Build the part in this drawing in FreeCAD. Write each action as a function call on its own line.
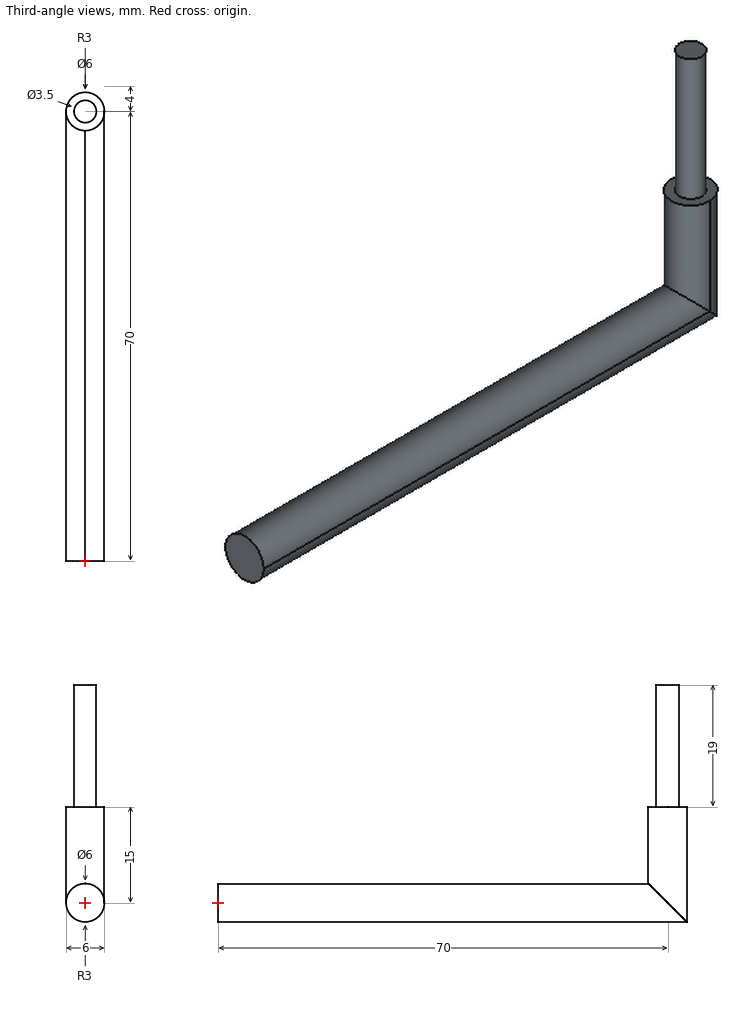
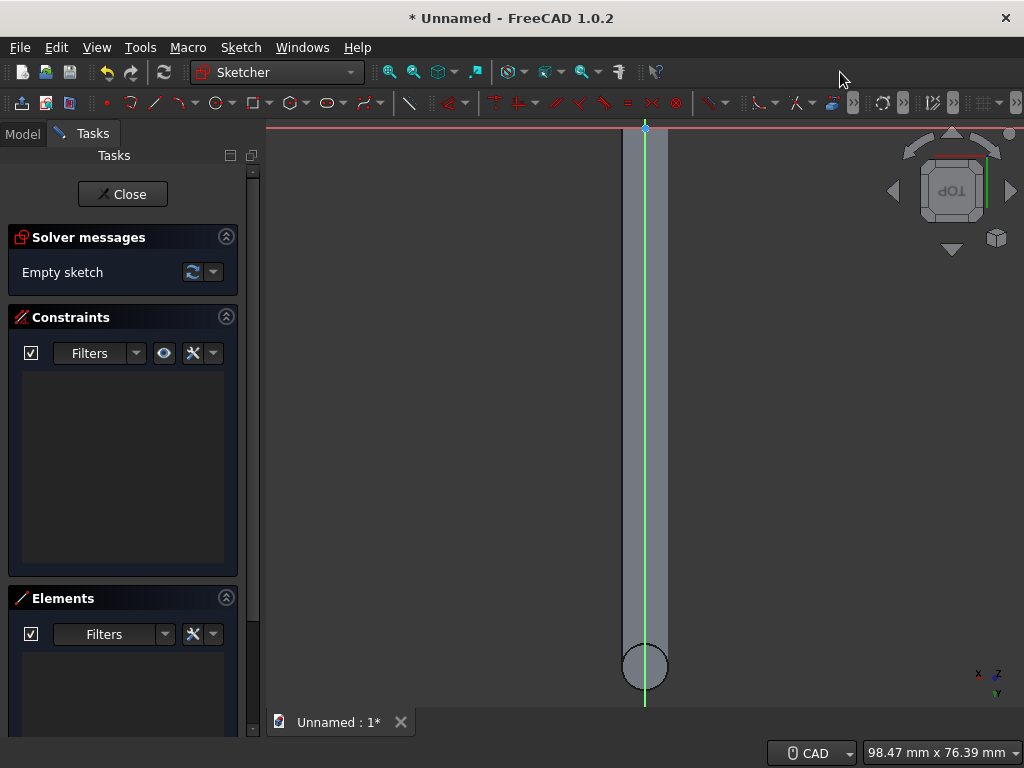
scroll(576, 413, down, 5)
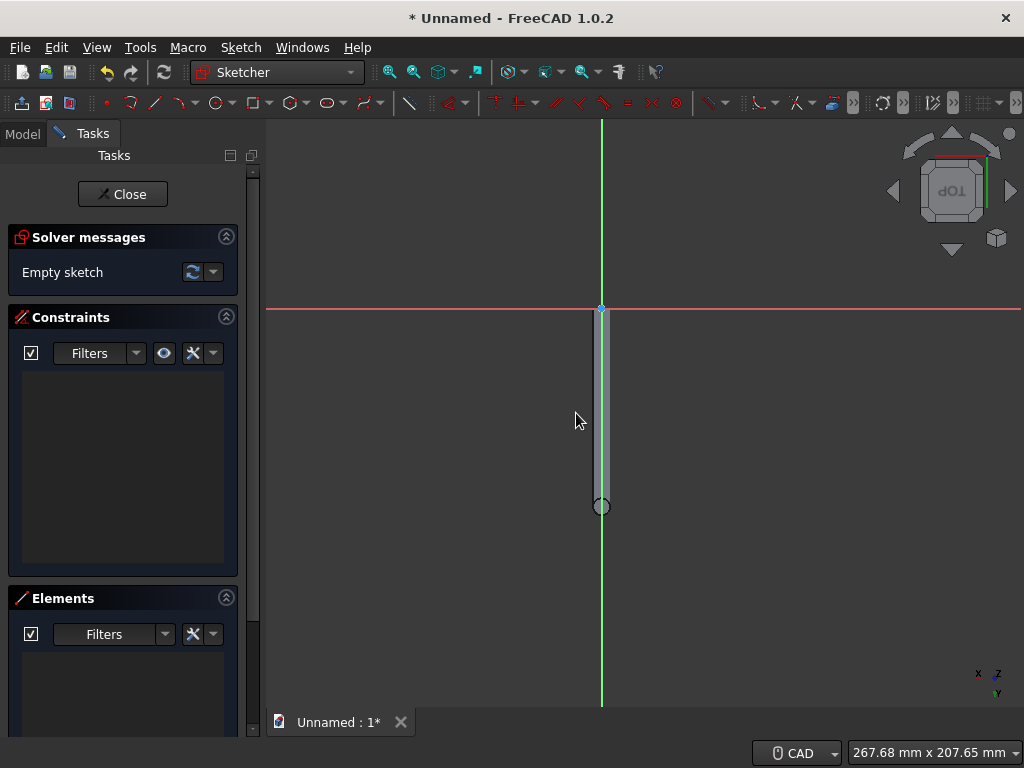
scroll(603, 512, up, 15)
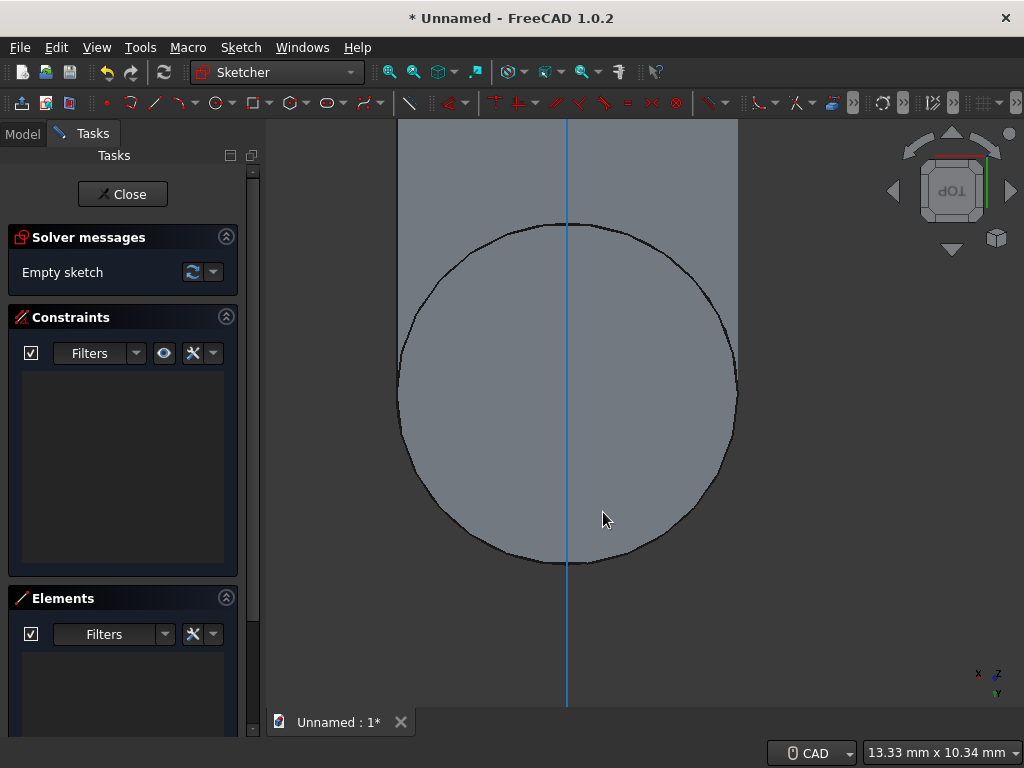
scroll(556, 371, up, 3)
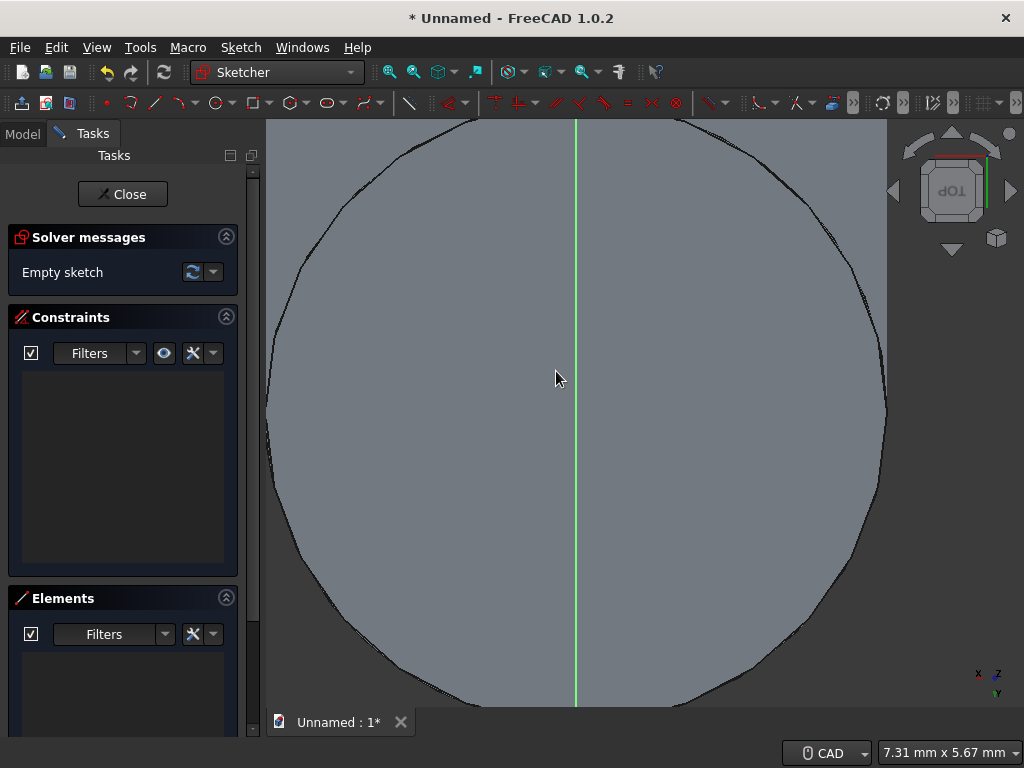
key(g)
key(c)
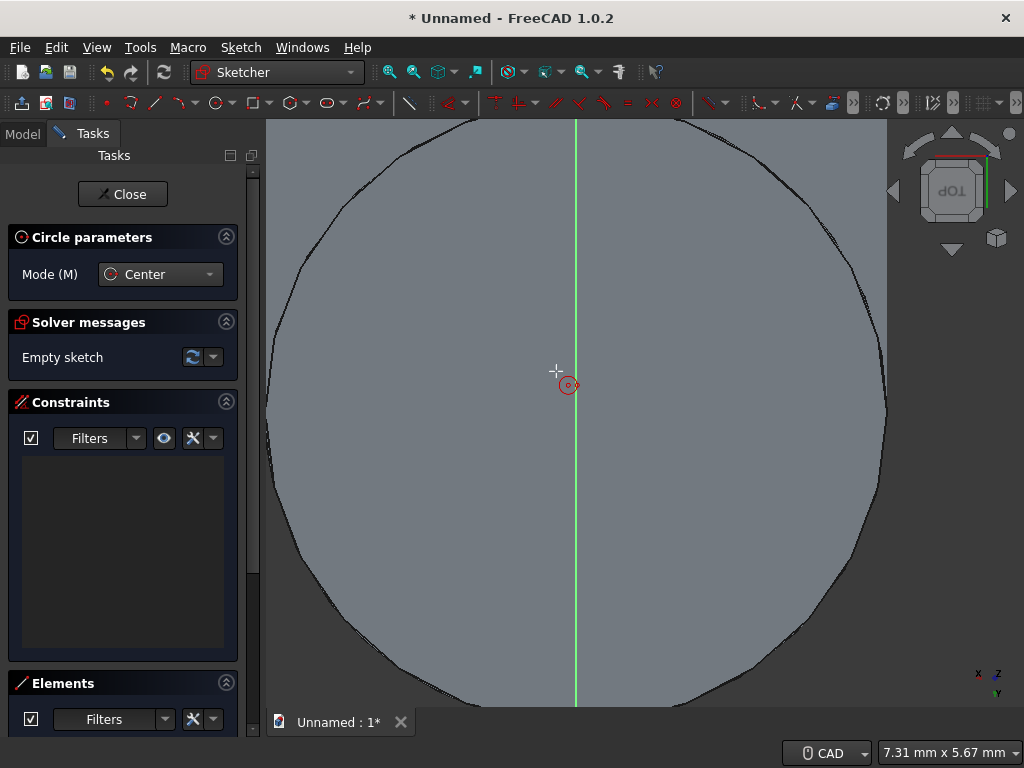
click(576, 413)
click(704, 284)
key(Escape)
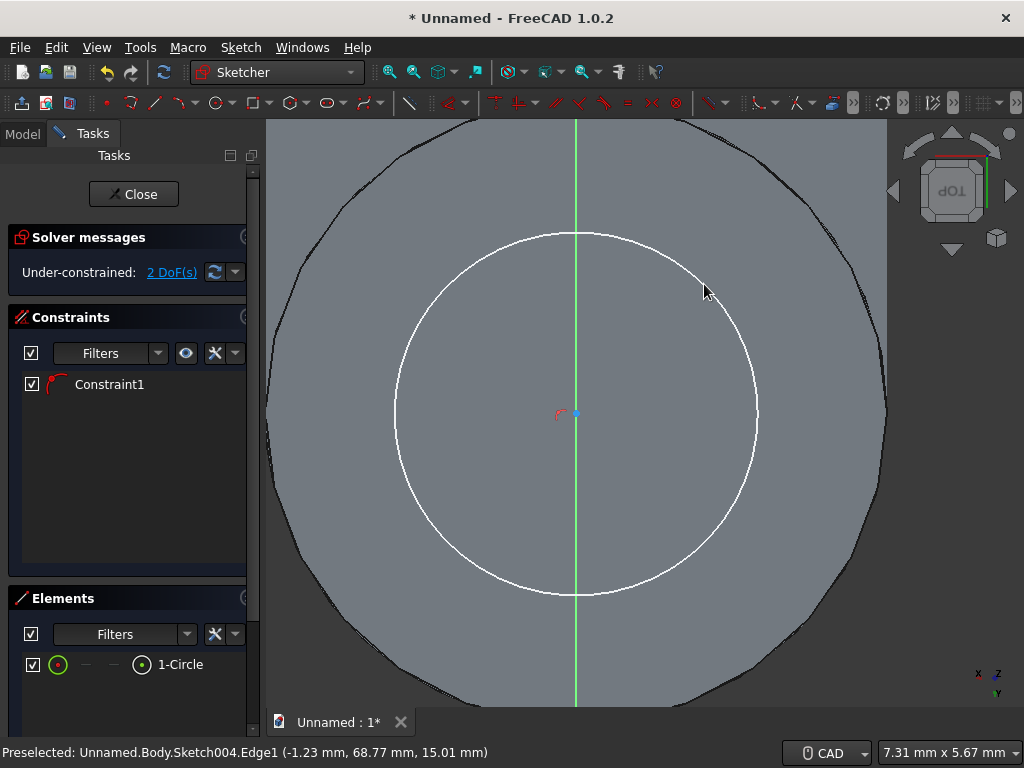
click(448, 104)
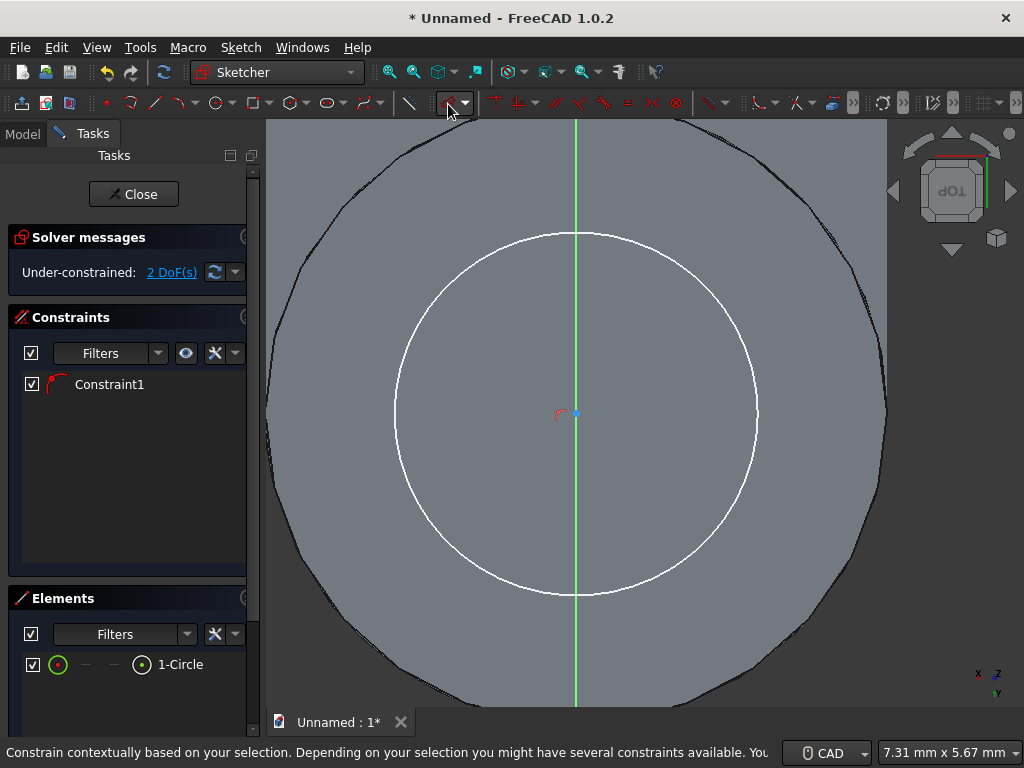
click(704, 285)
click(727, 262)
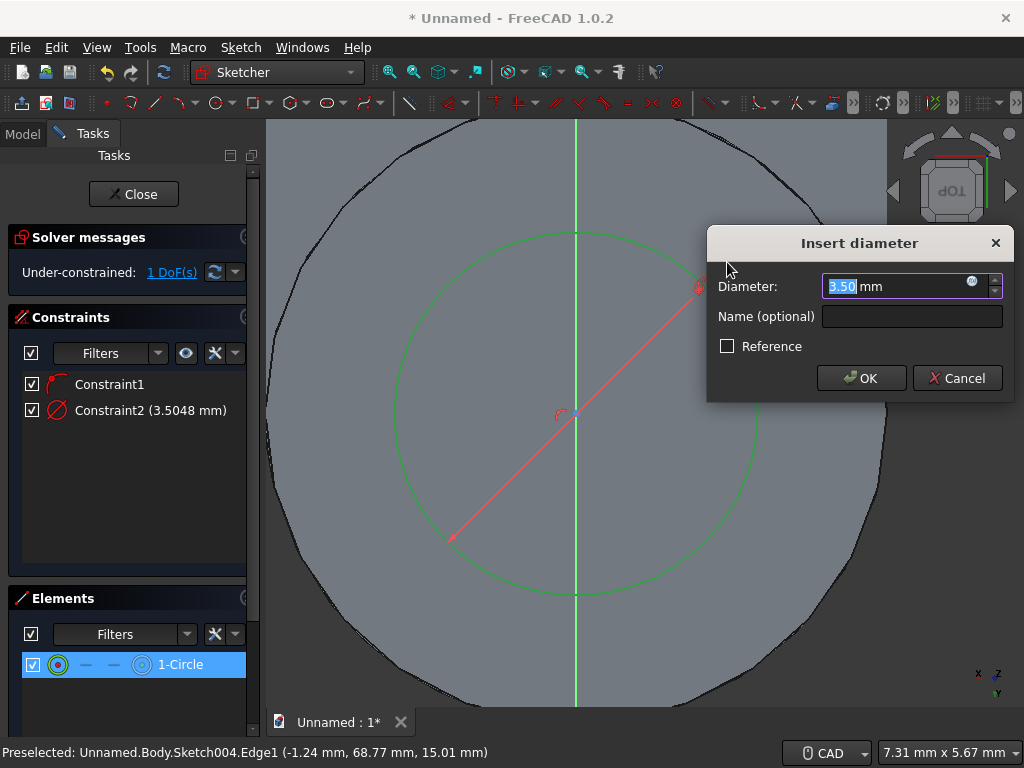
text(3.5)
key(Return)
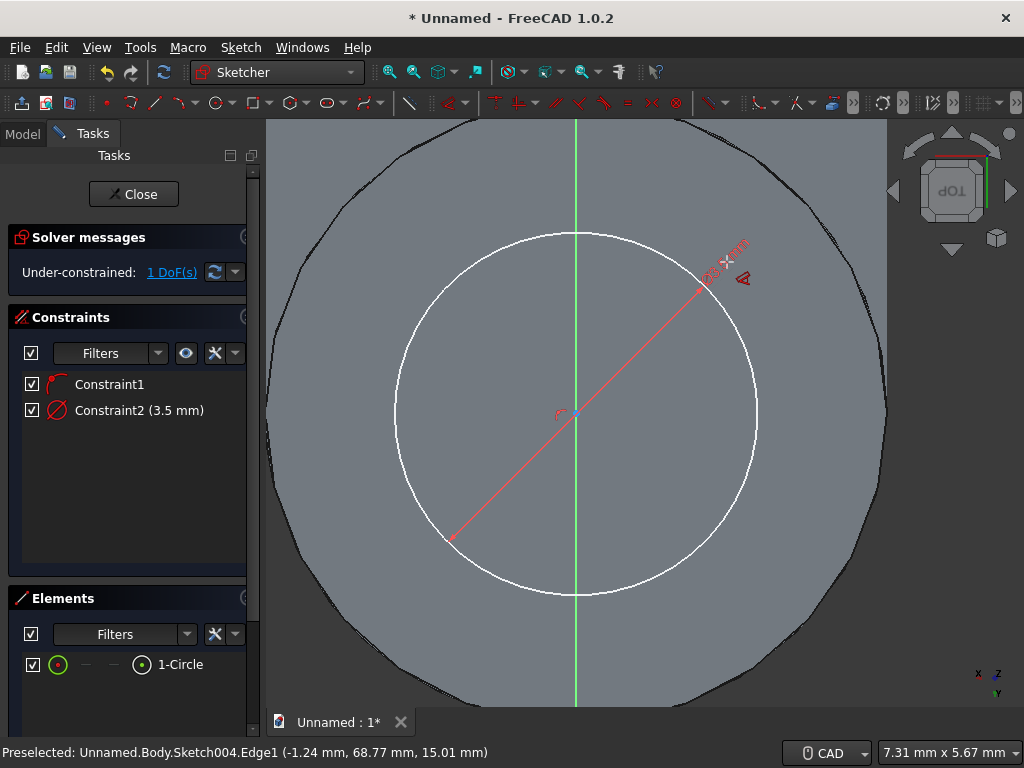
click(576, 414)
click(610, 281)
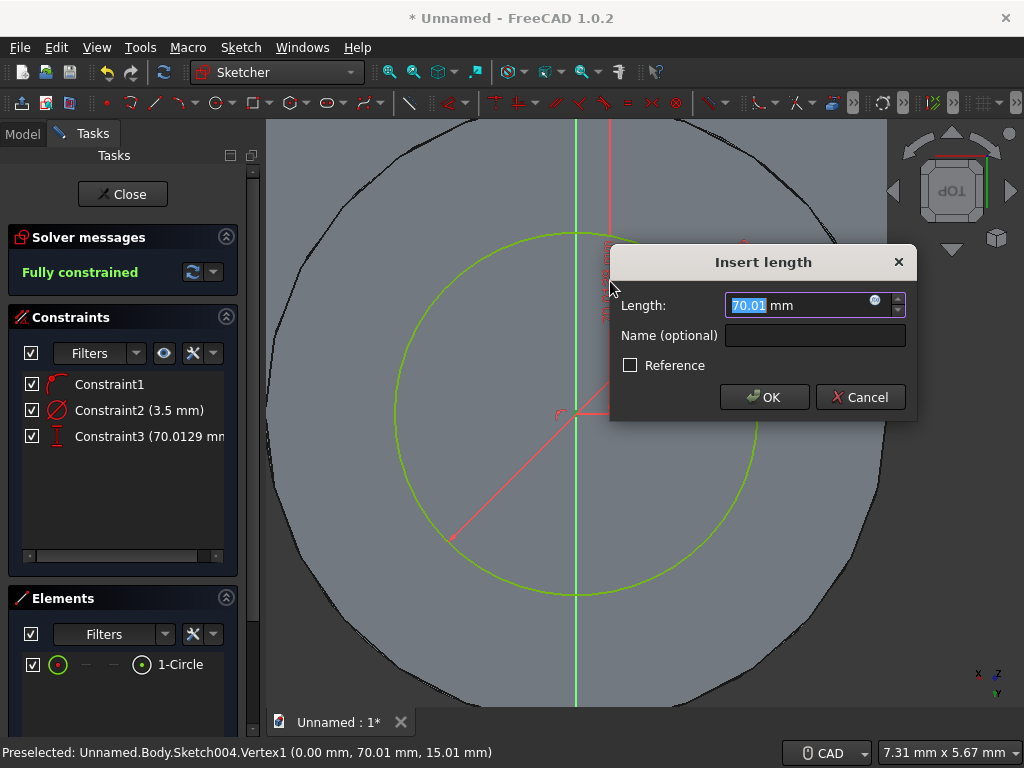
text(70)
key(Return)
key(Escape)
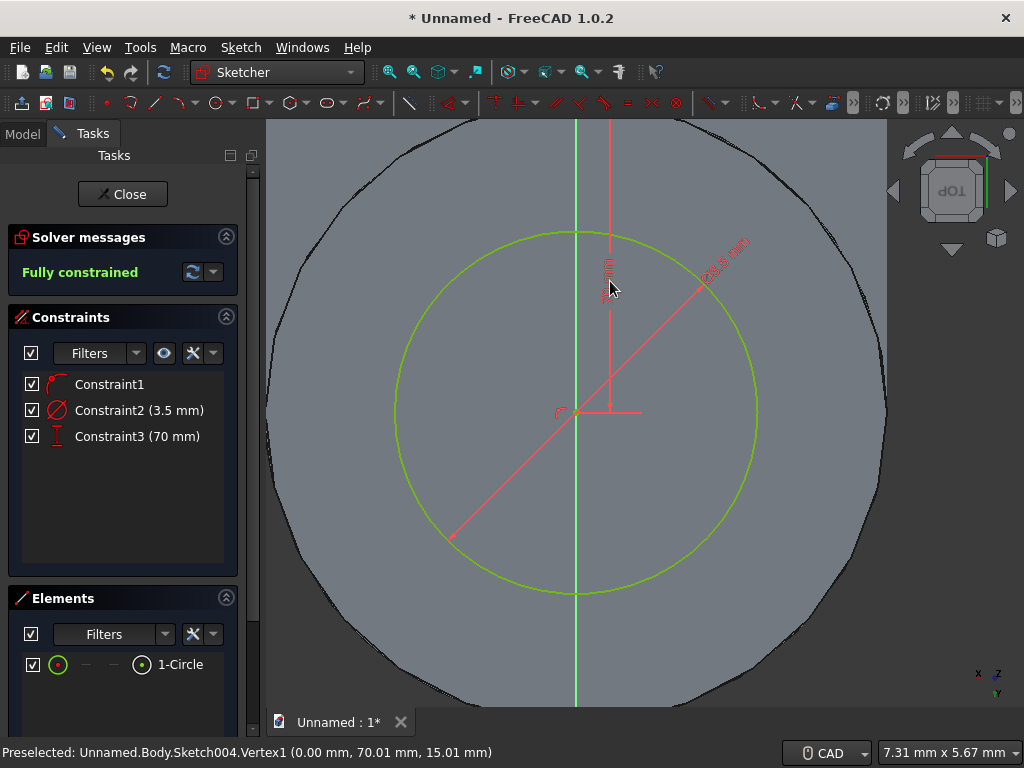
click(123, 194)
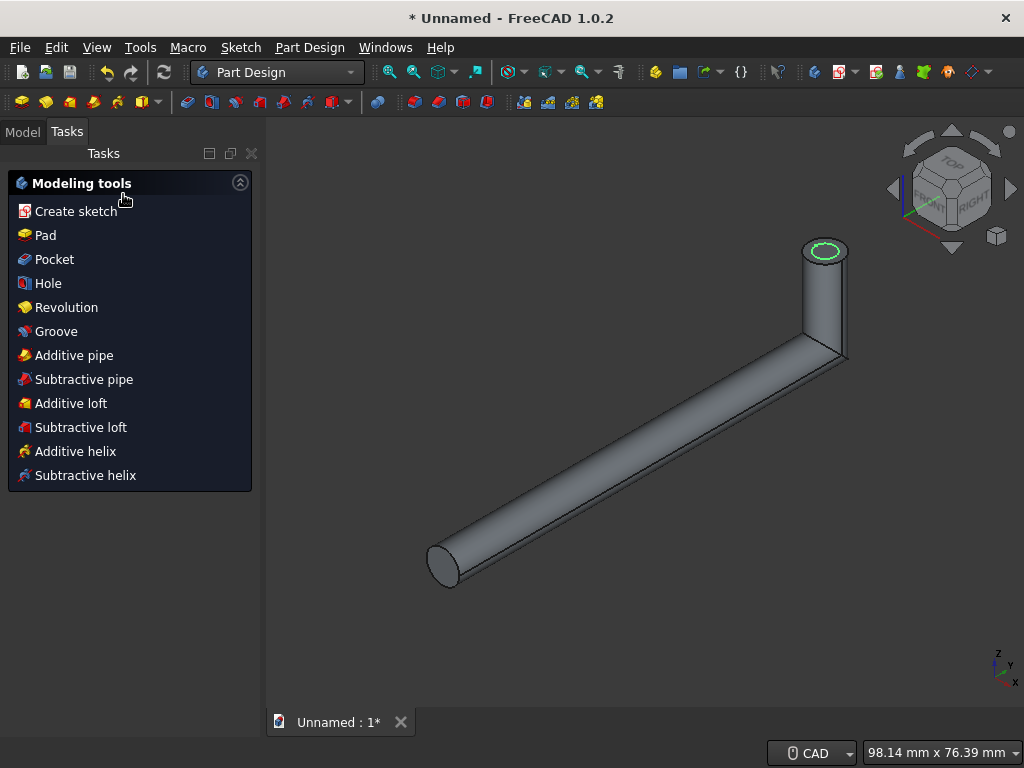
click(22, 102)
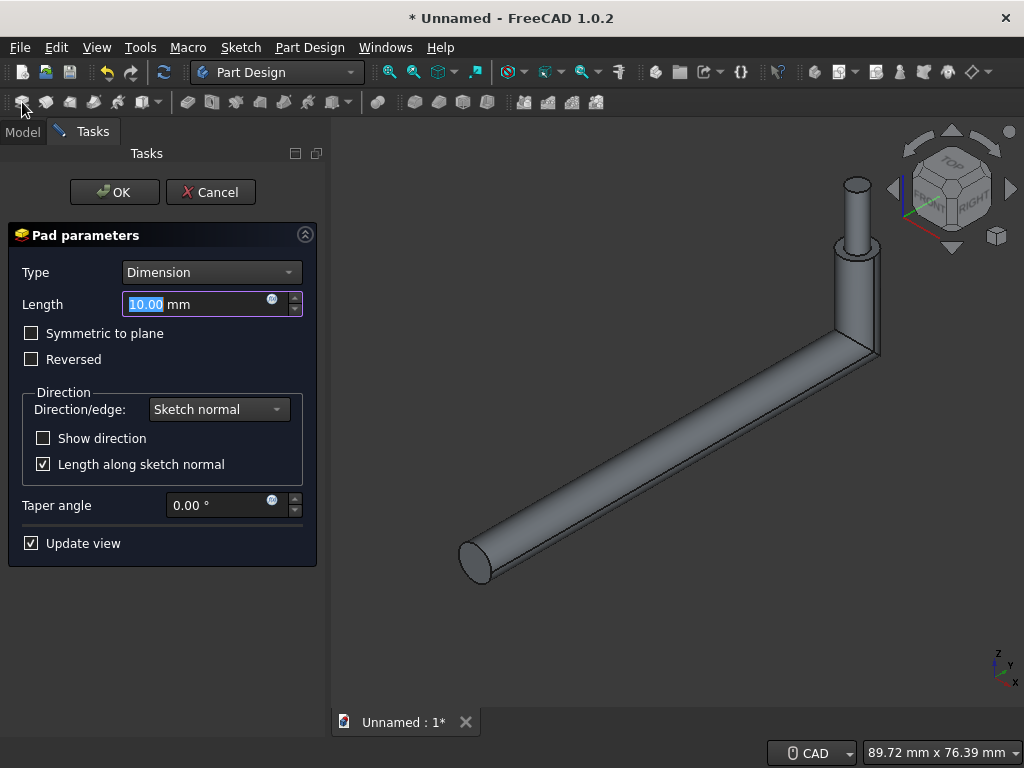
text(19)
key(Tab)